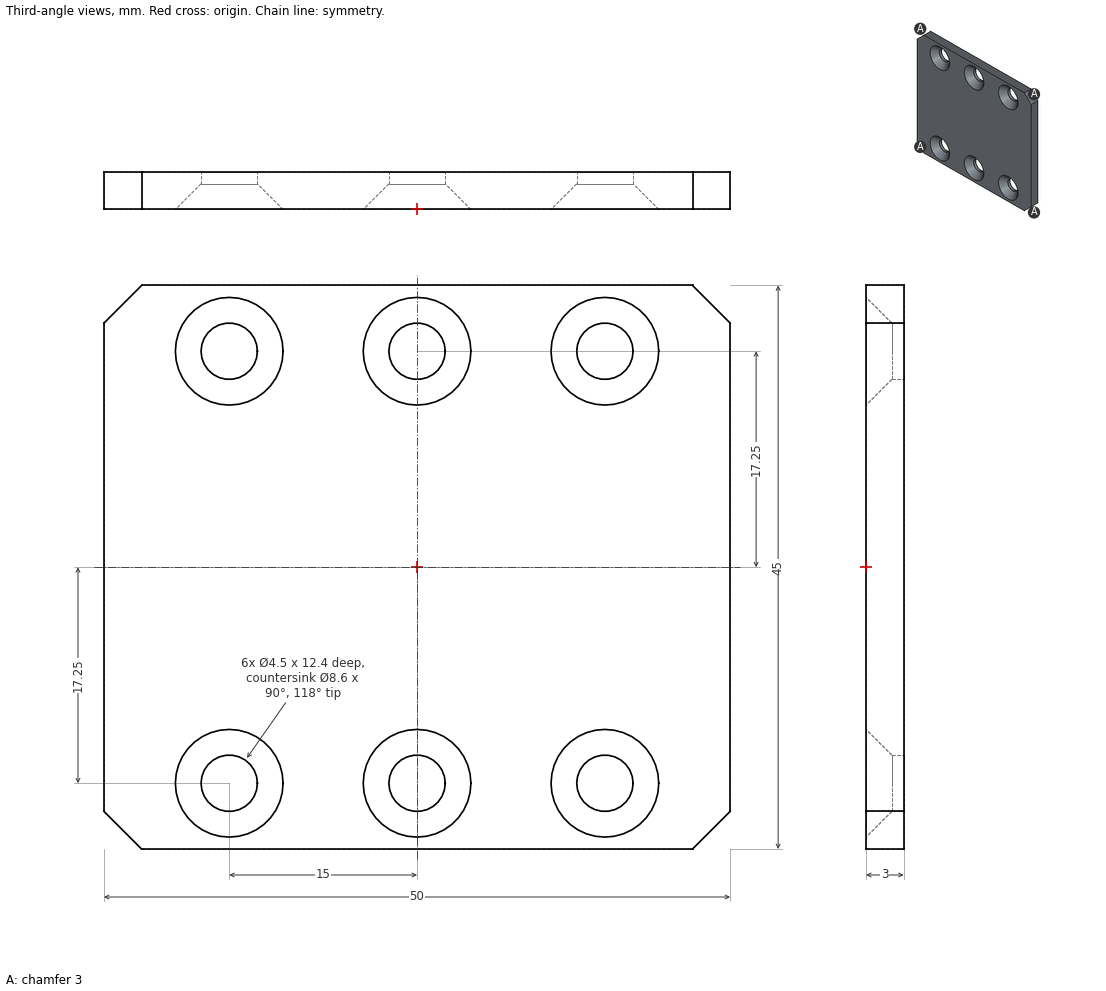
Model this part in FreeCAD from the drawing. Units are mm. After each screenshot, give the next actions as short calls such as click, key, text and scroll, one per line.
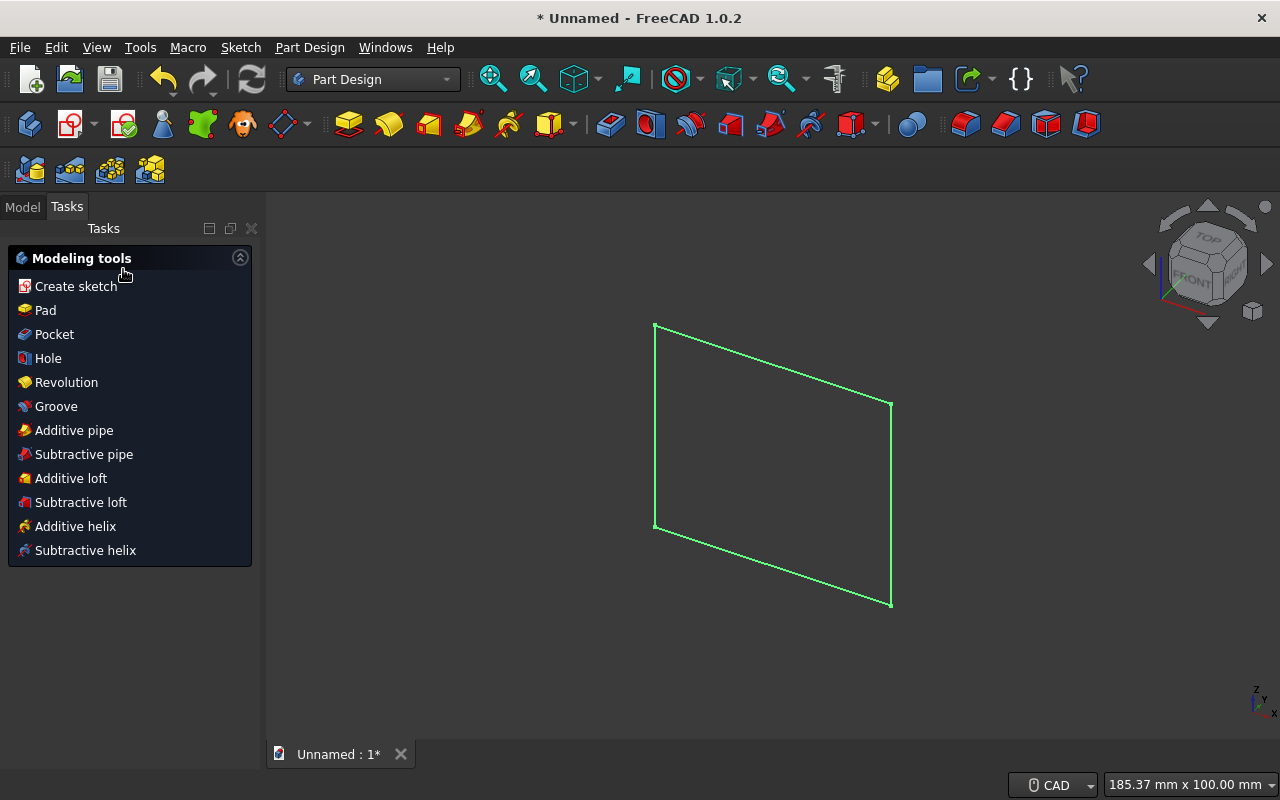
click(350, 124)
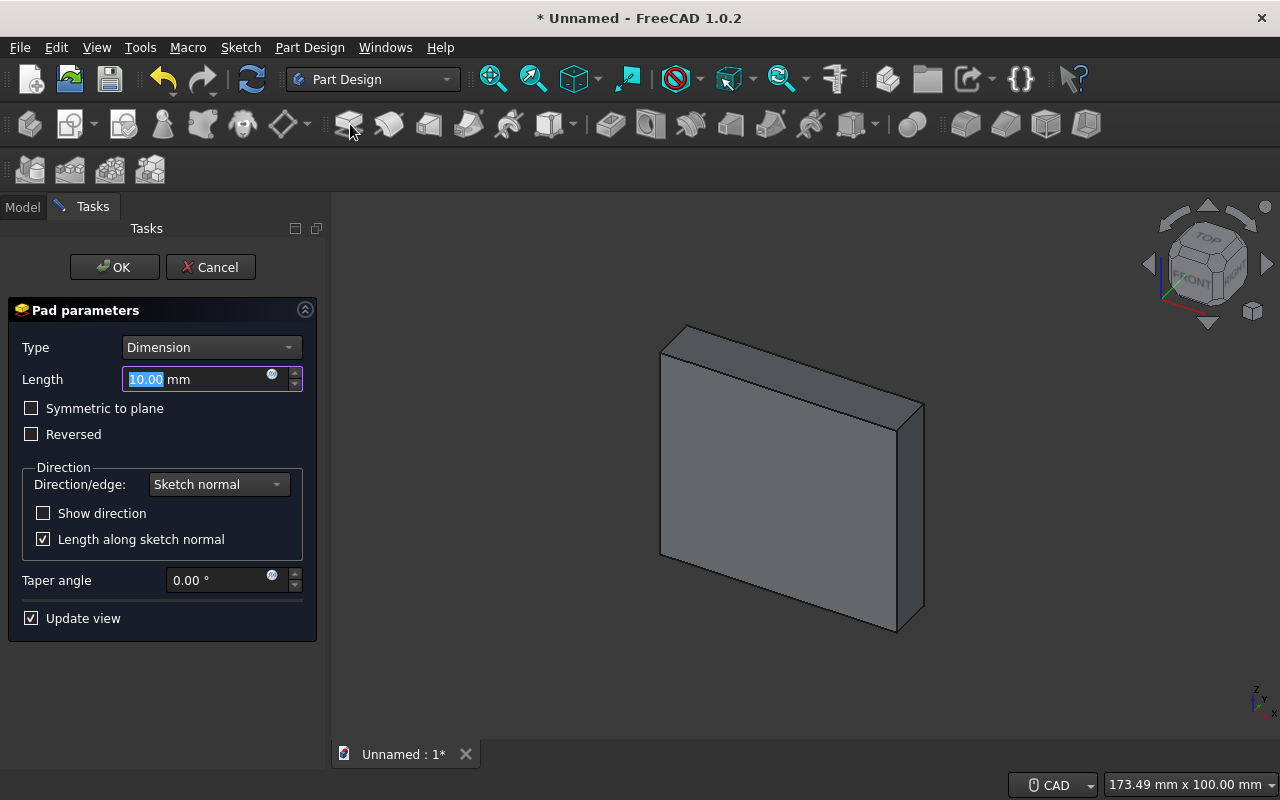
text(3)
key(Tab)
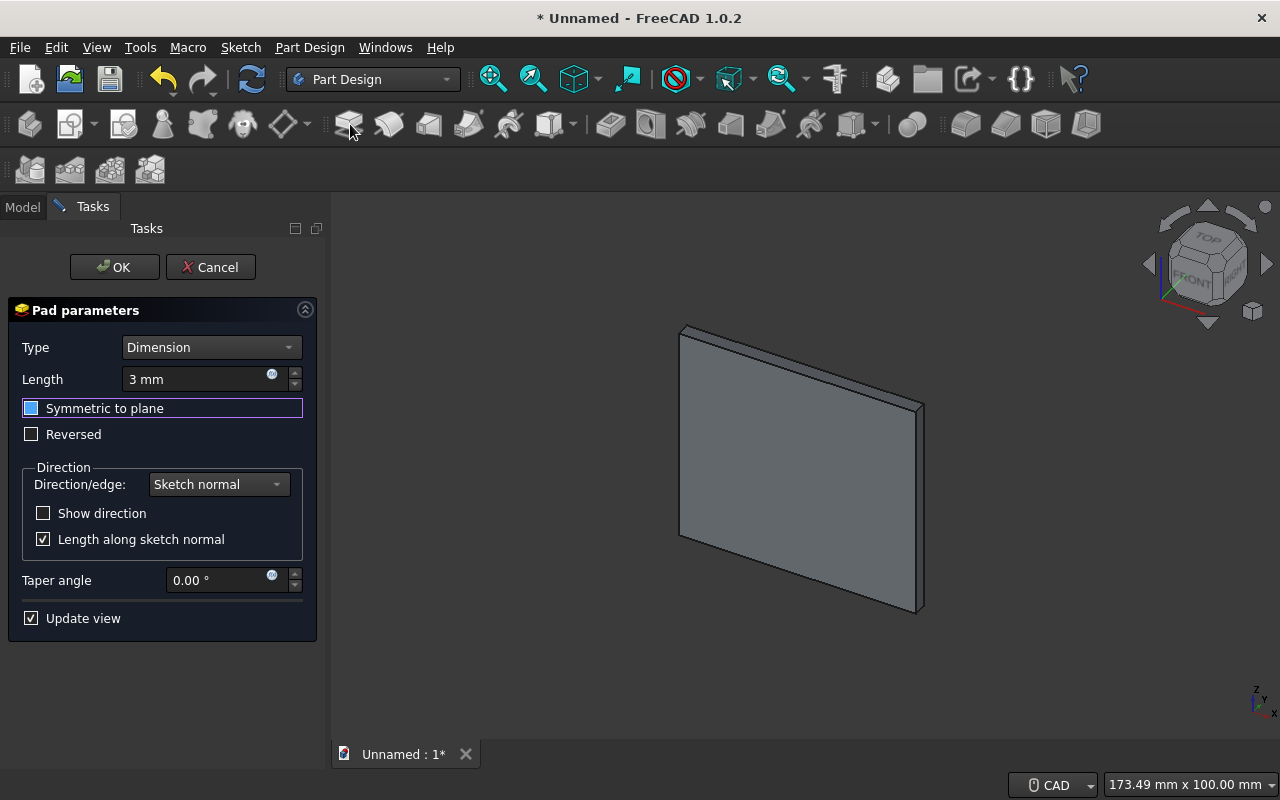
click(30, 434)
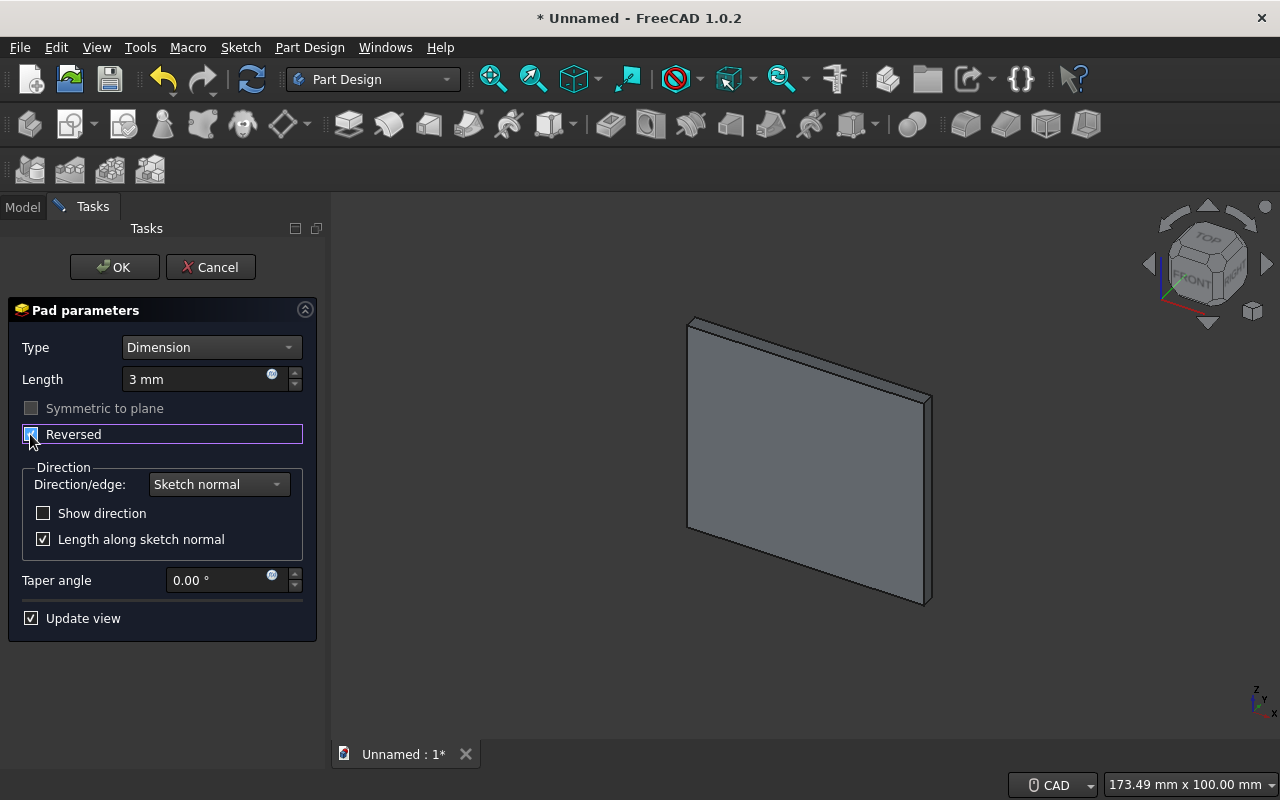
click(115, 267)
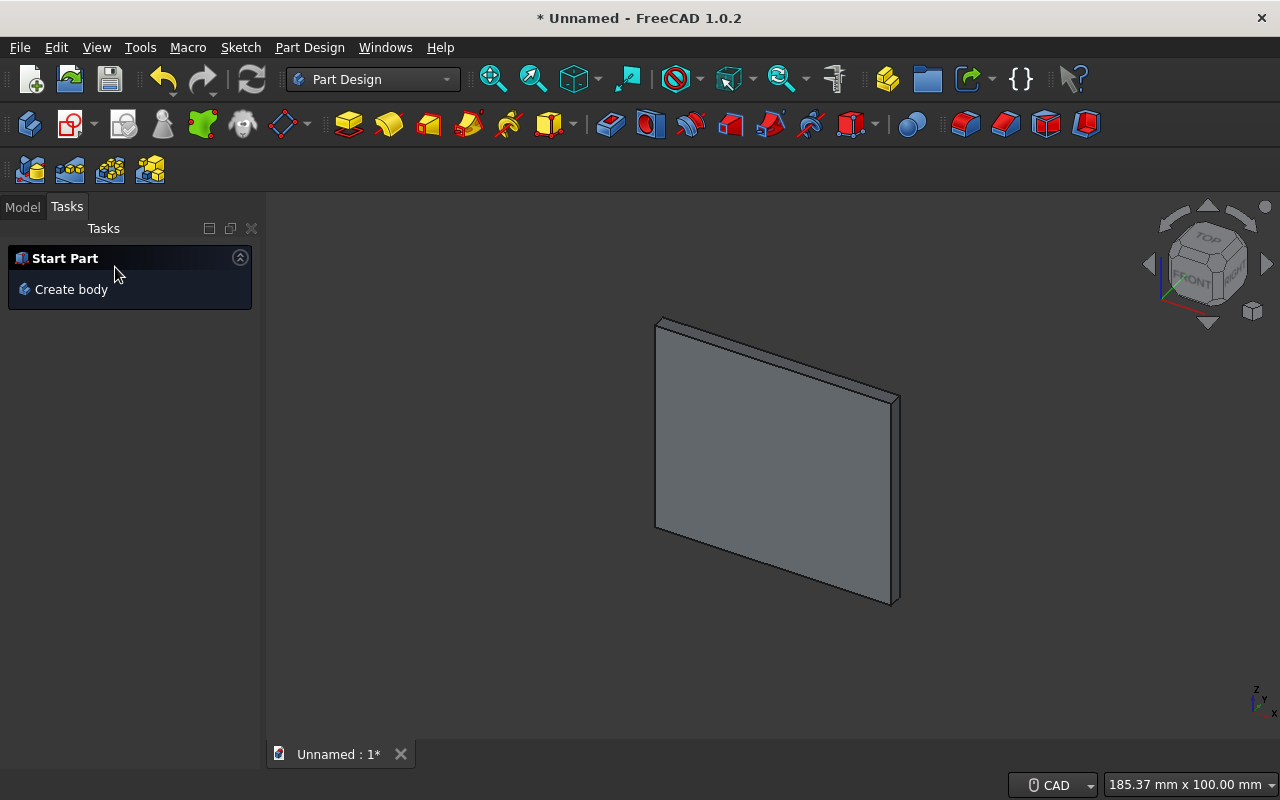
click(70, 124)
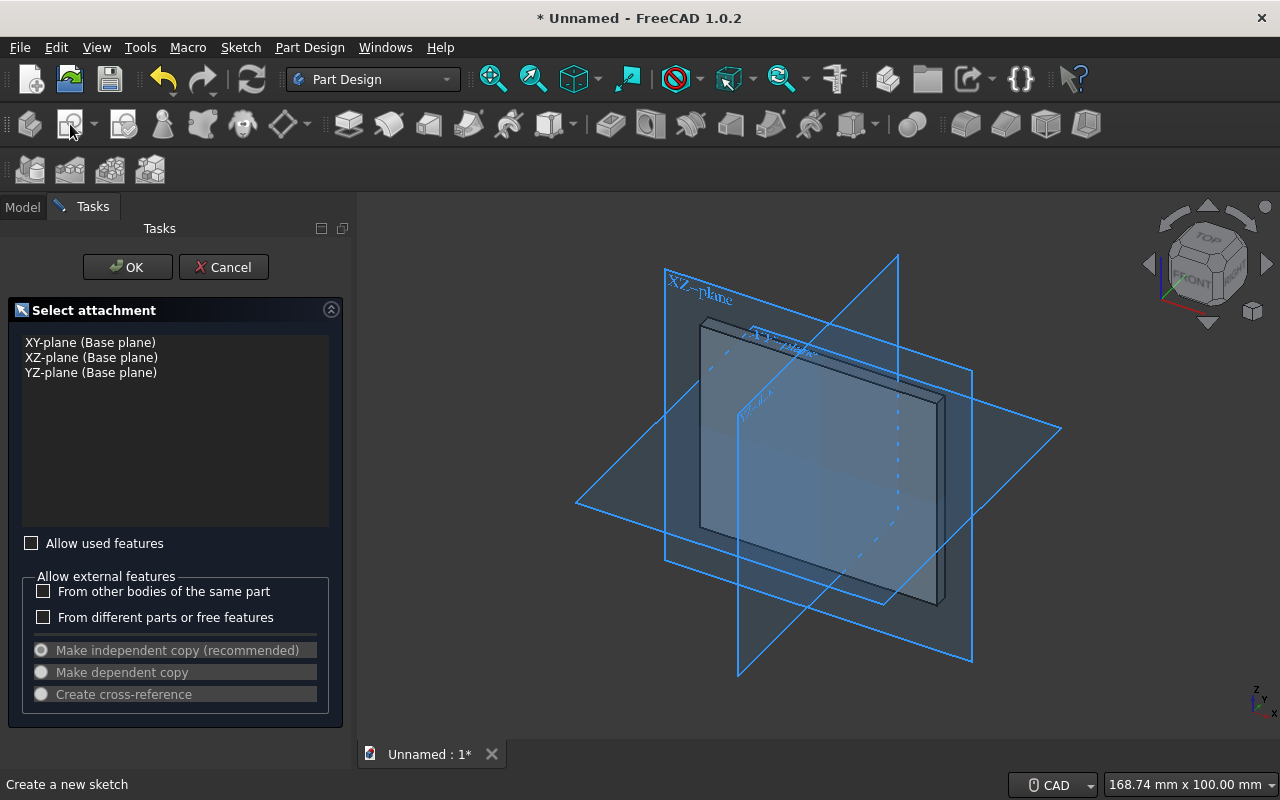
click(82, 358)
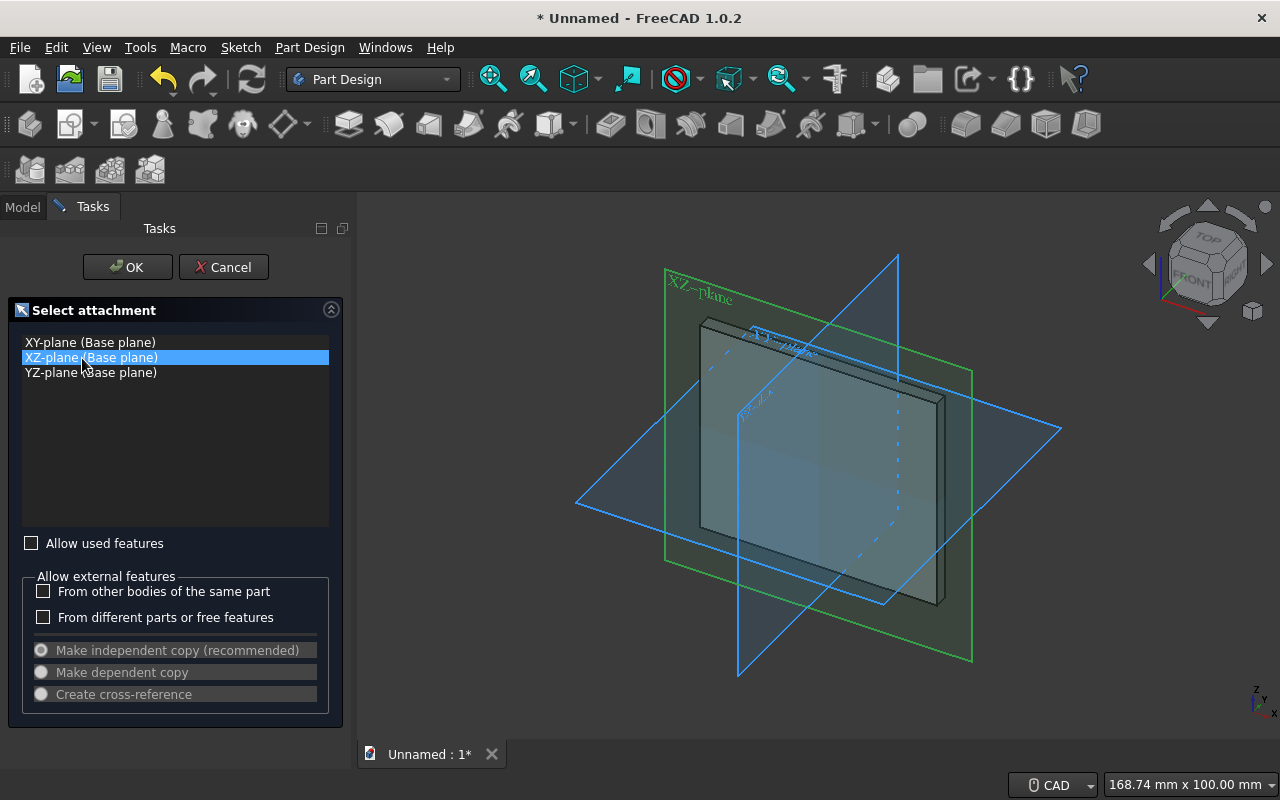
click(128, 267)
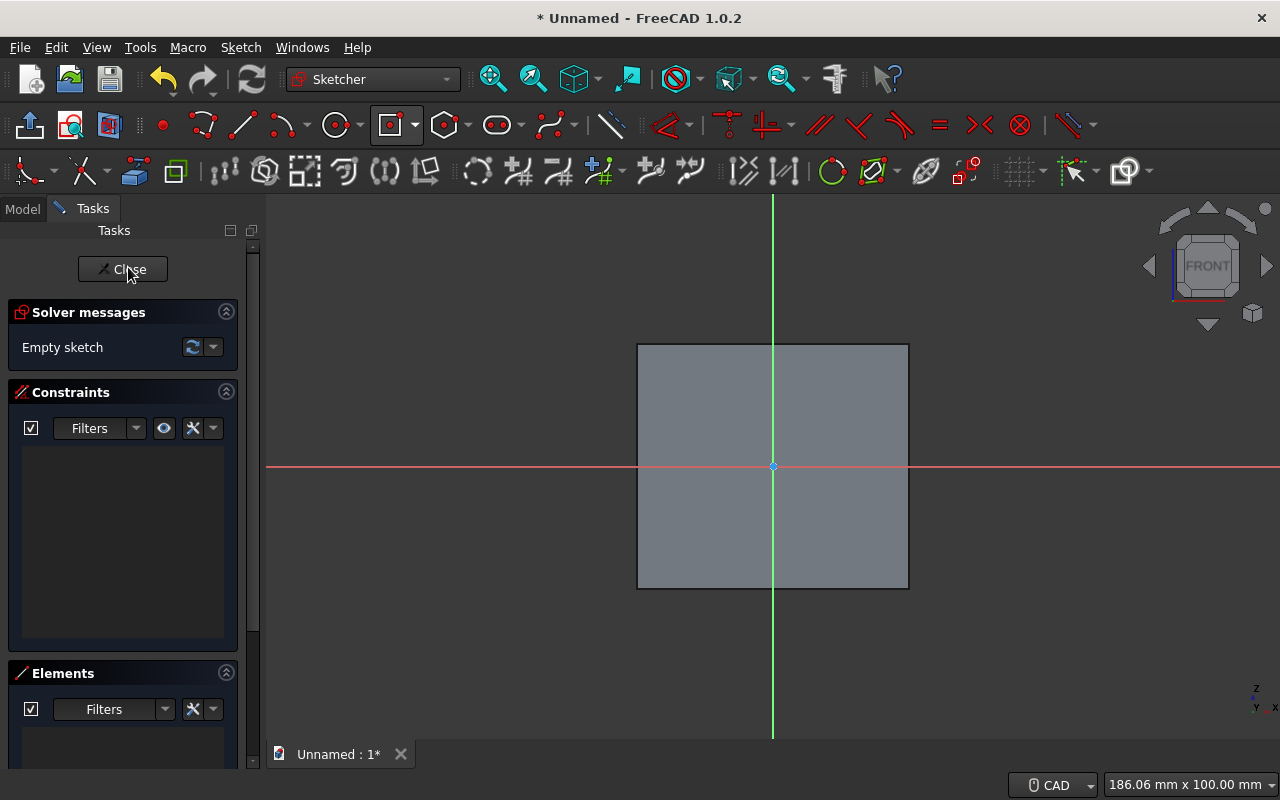
scroll(912, 467, up, 2)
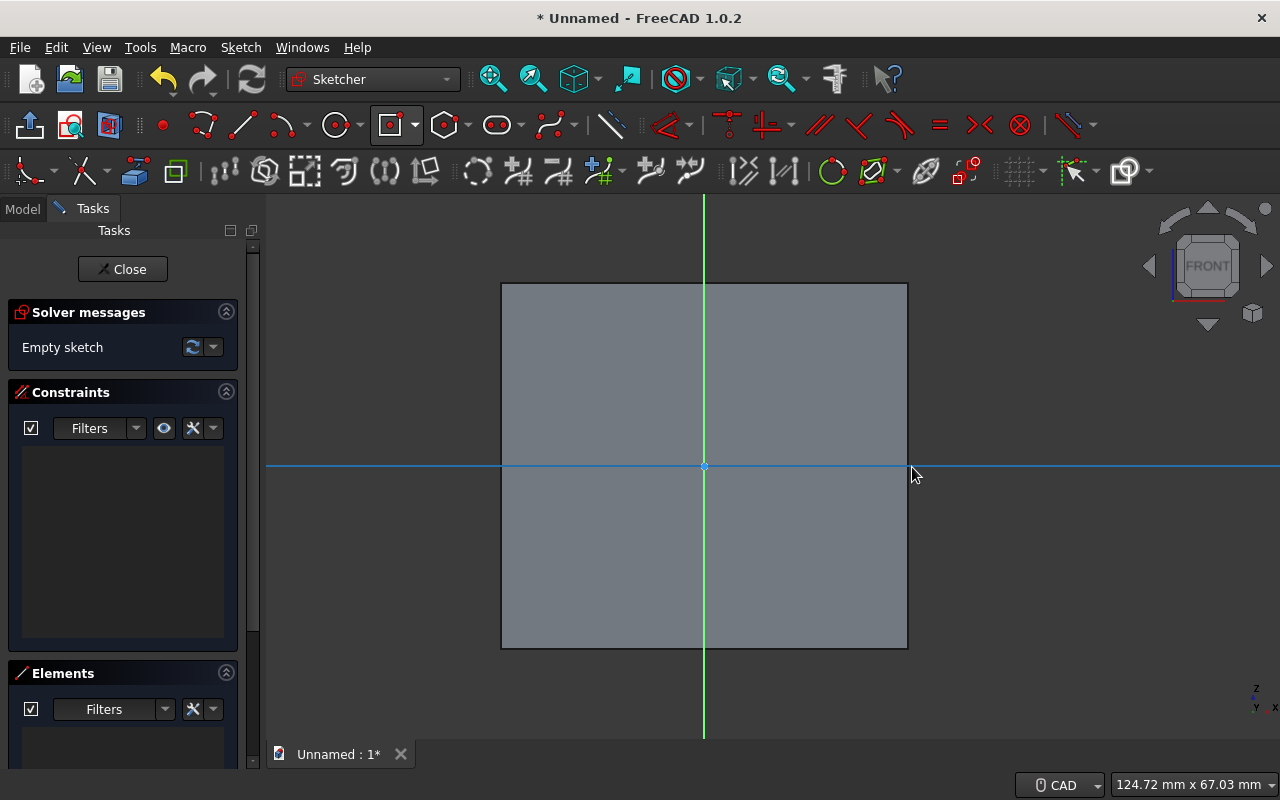
click(336, 126)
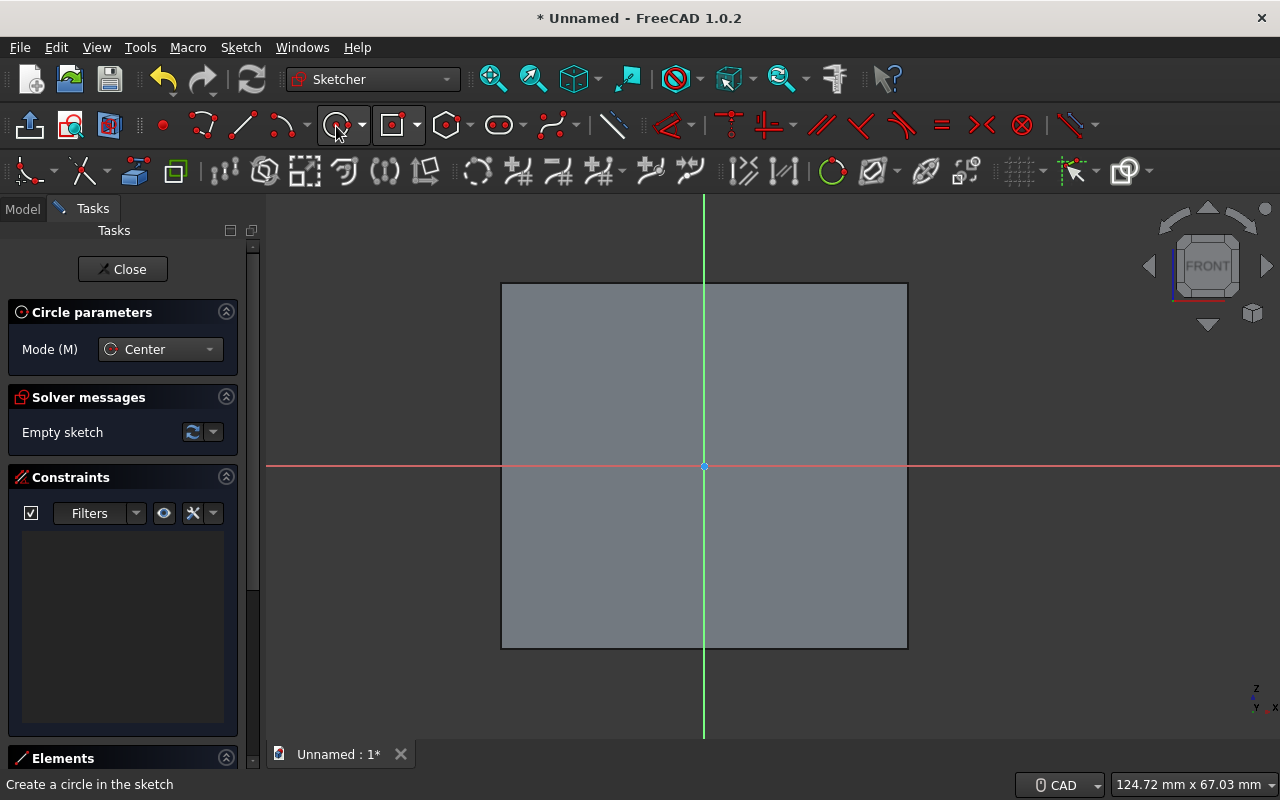
scroll(582, 606, up, 2)